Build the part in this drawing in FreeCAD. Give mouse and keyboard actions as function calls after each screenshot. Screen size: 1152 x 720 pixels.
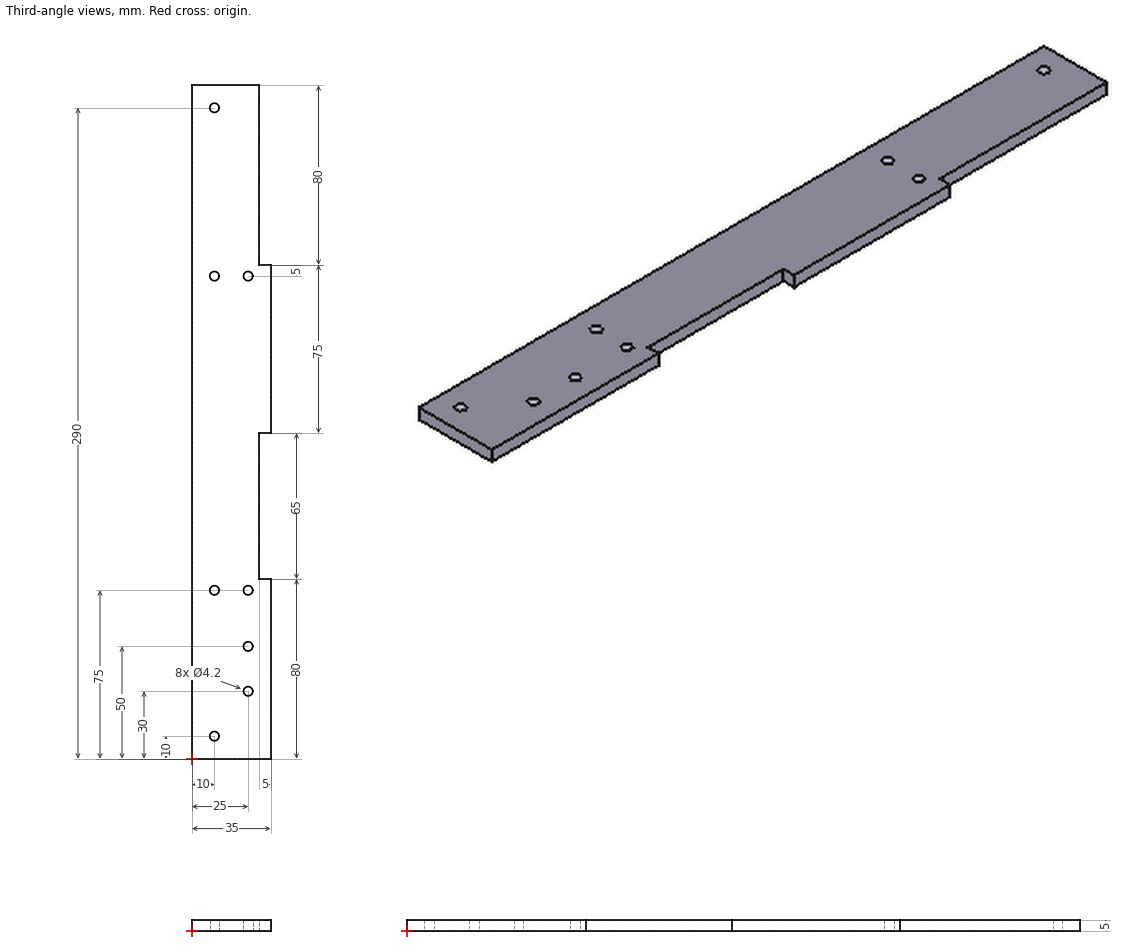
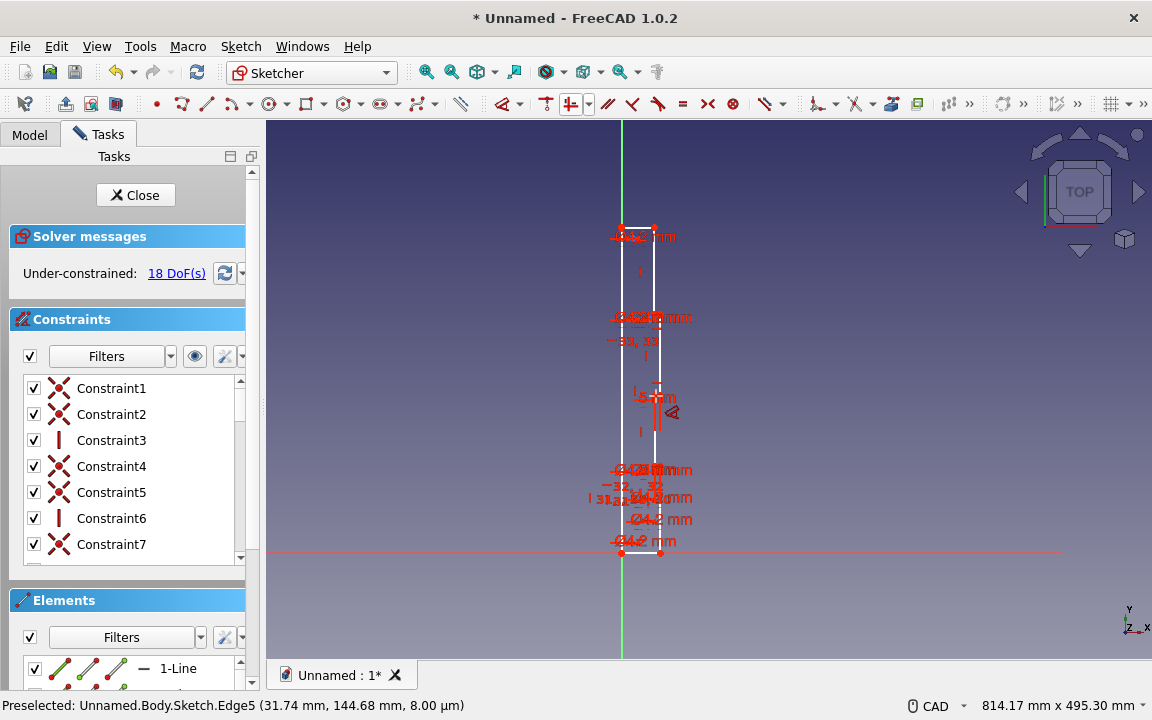
scroll(658, 315, up, 11)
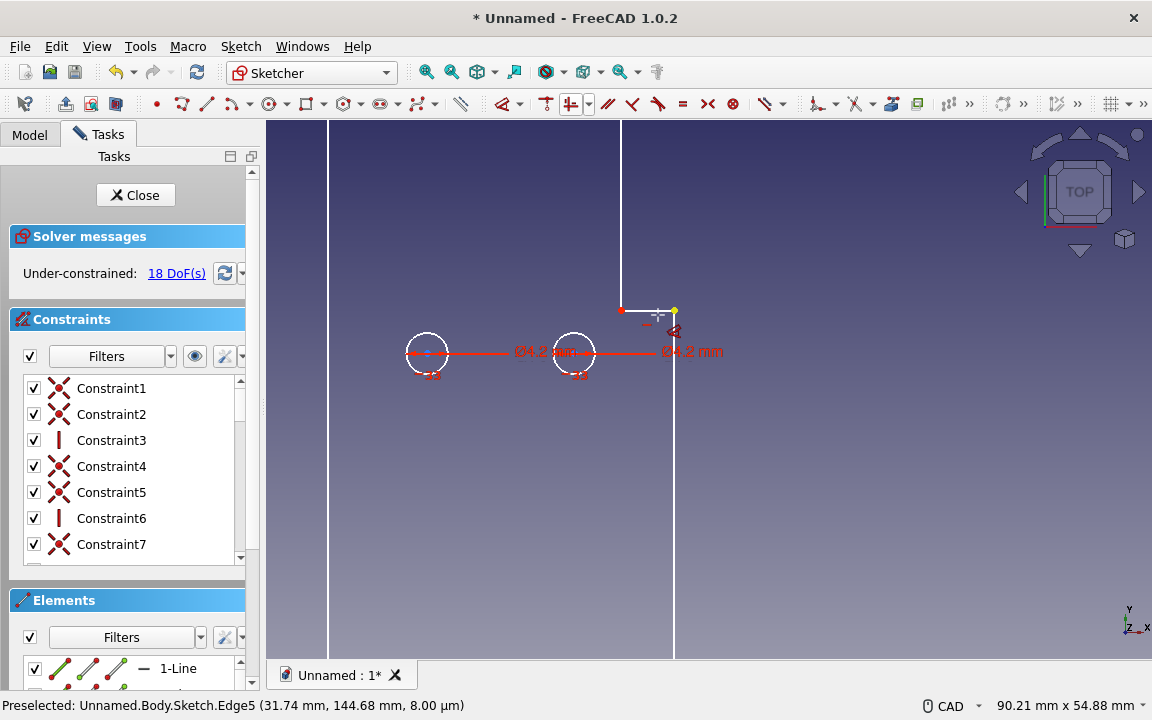
click(658, 311)
click(648, 277)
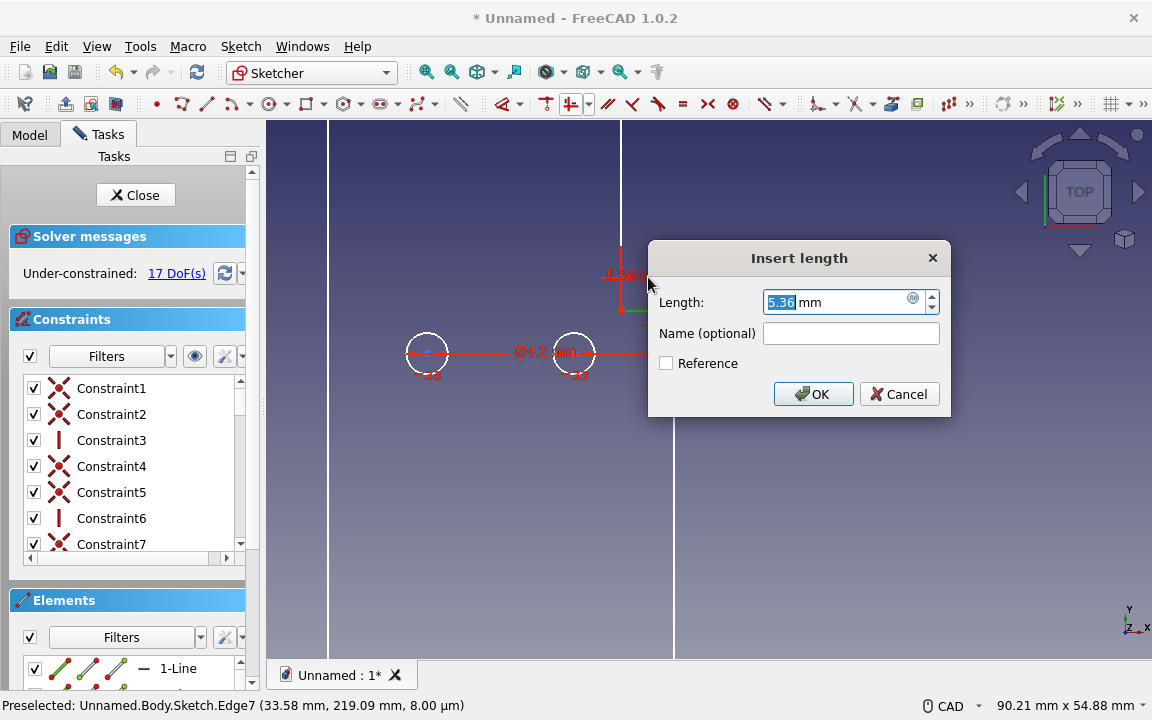
text(5)
key(Return)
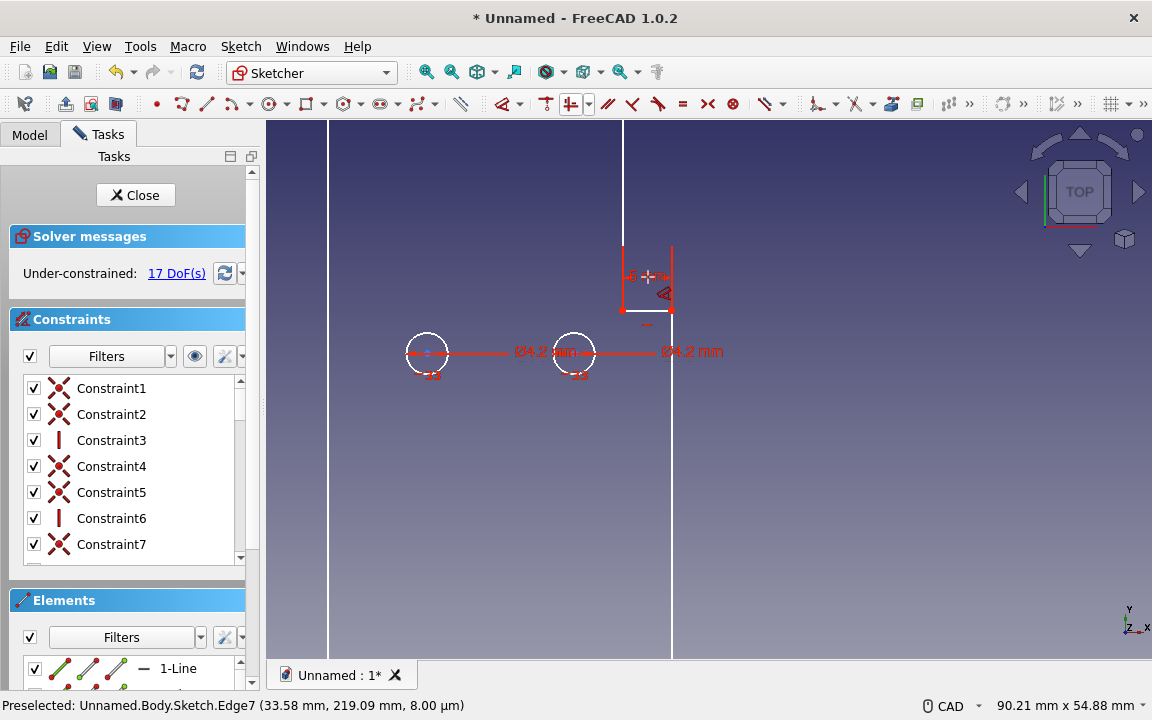
scroll(658, 315, down, 11)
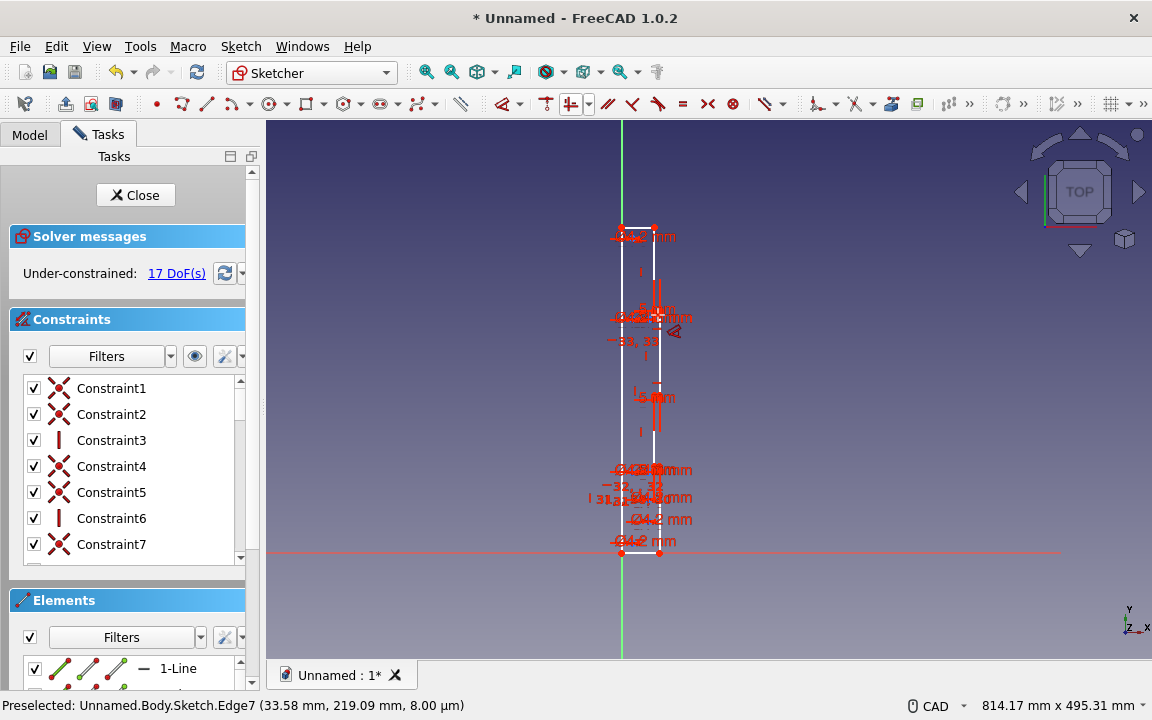
scroll(633, 553, up, 3)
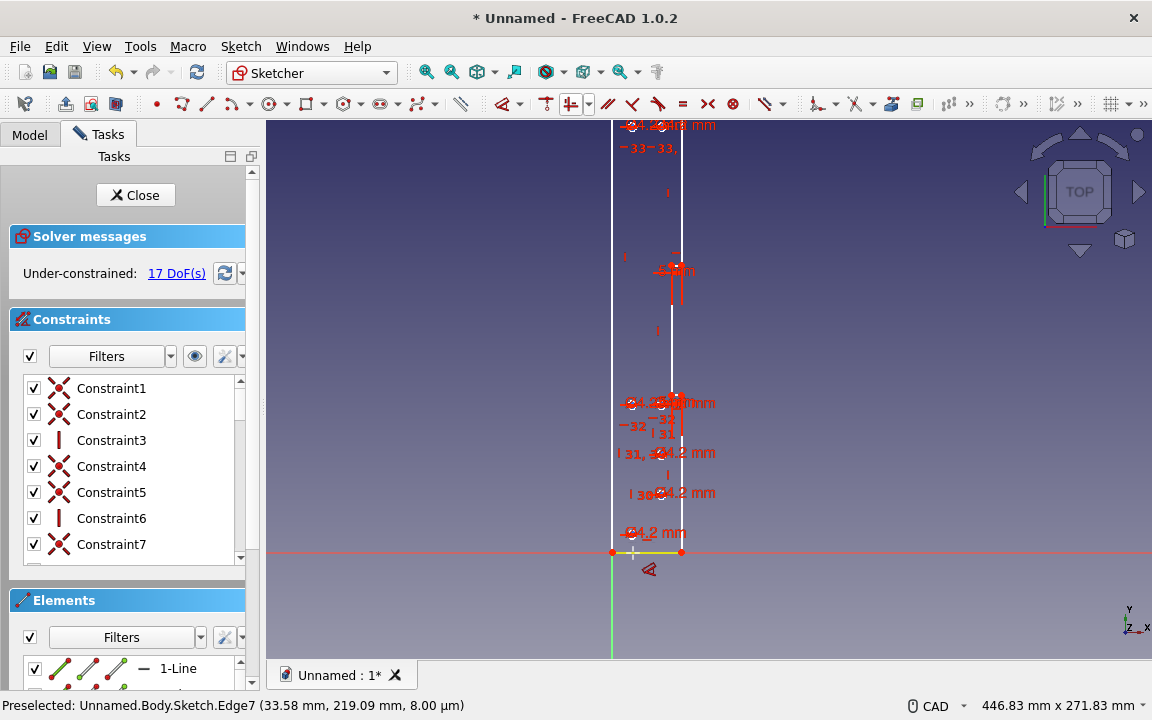
click(633, 553)
click(647, 587)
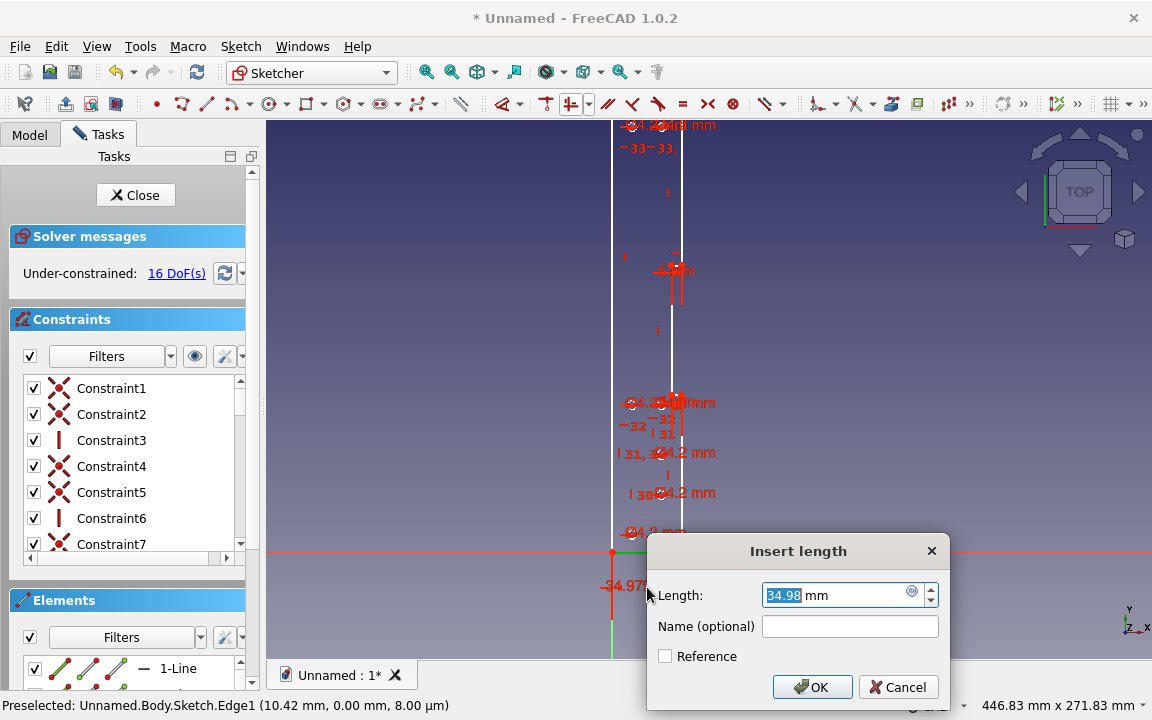
text(35)
key(Return)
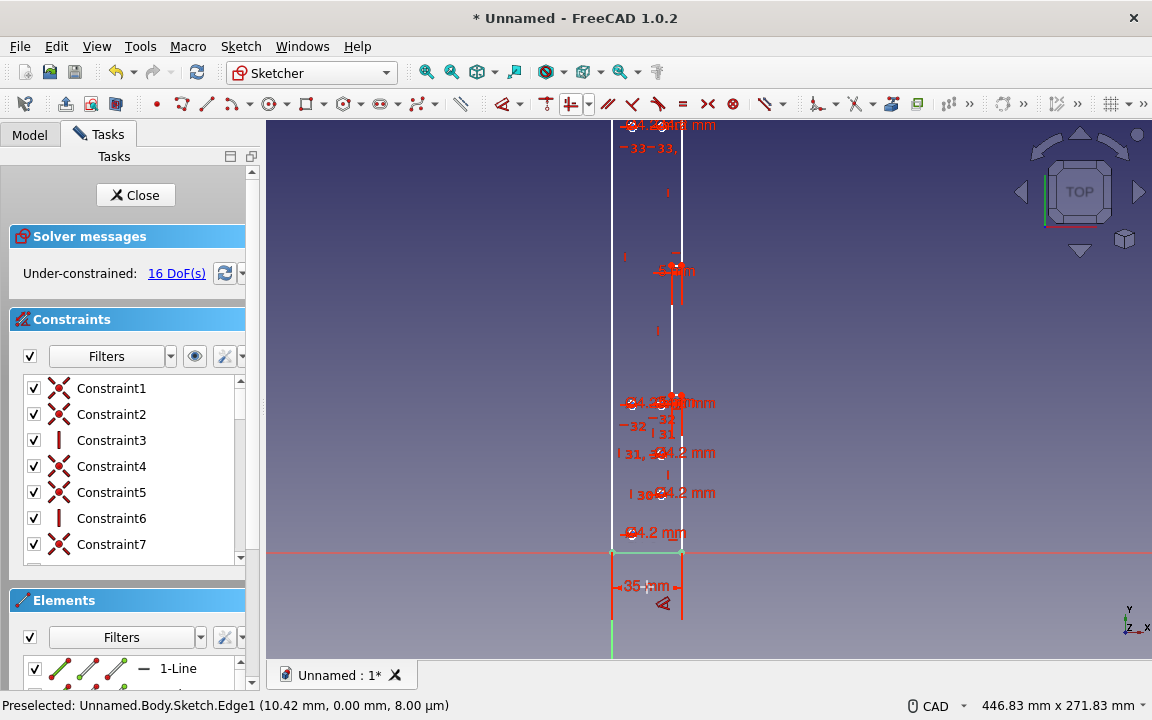
click(682, 506)
click(716, 474)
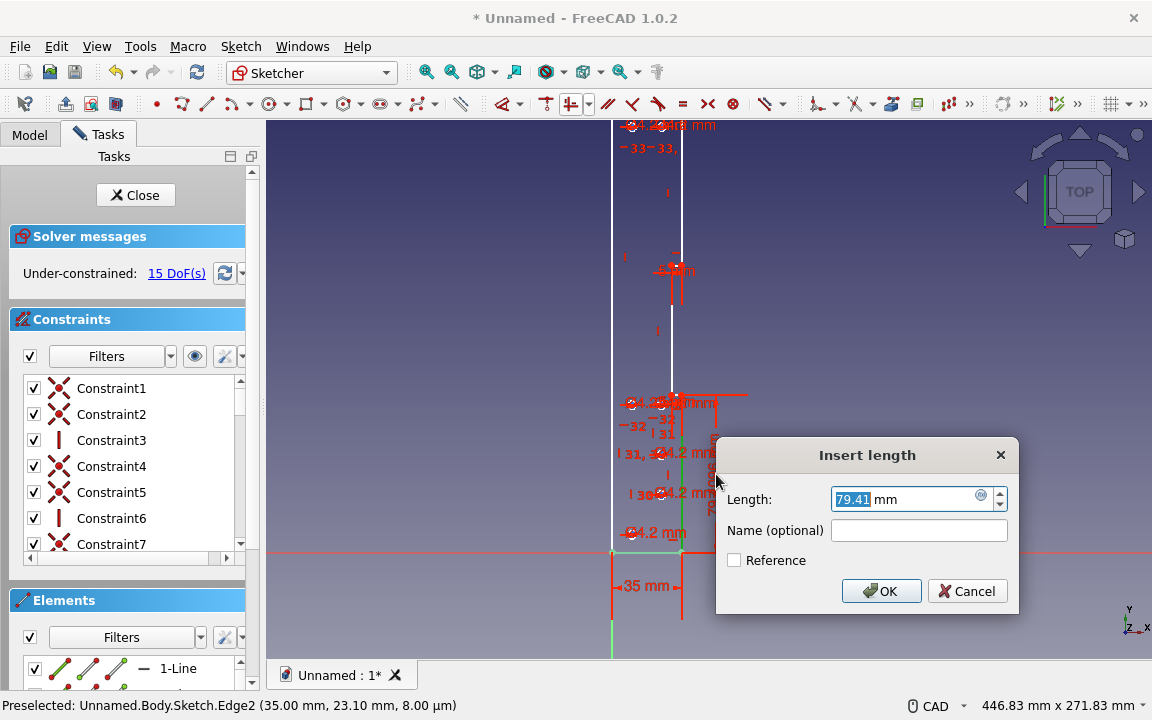
text(80)
key(Return)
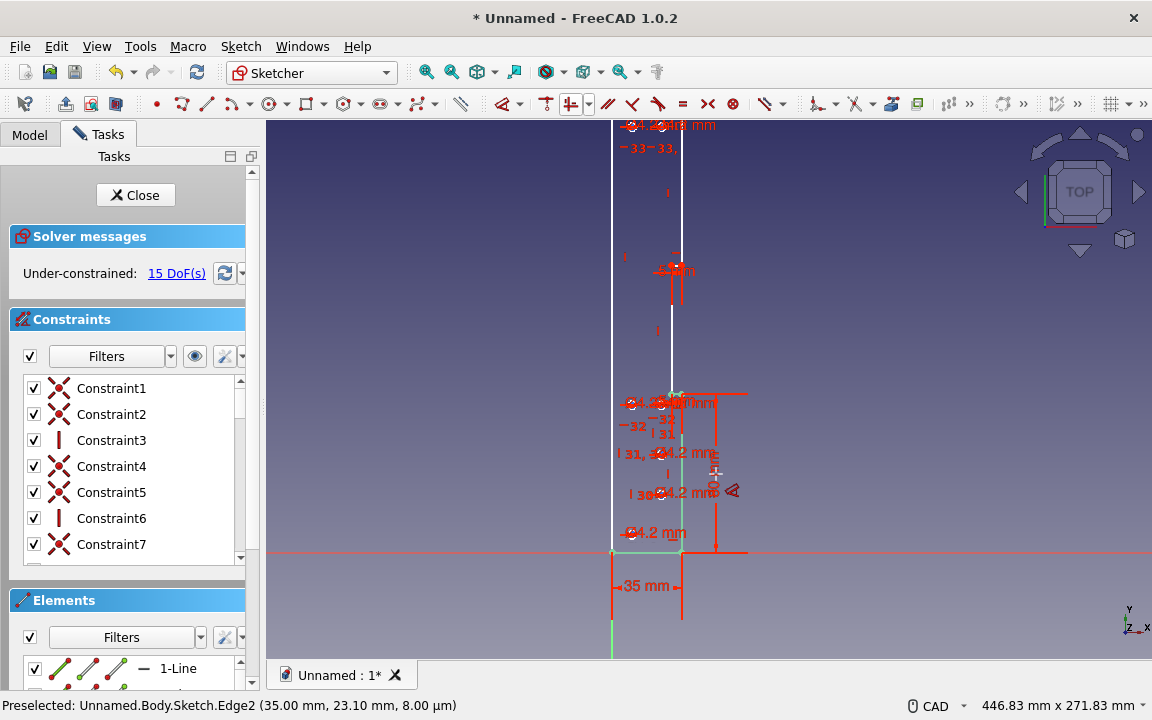
click(672, 356)
click(706, 330)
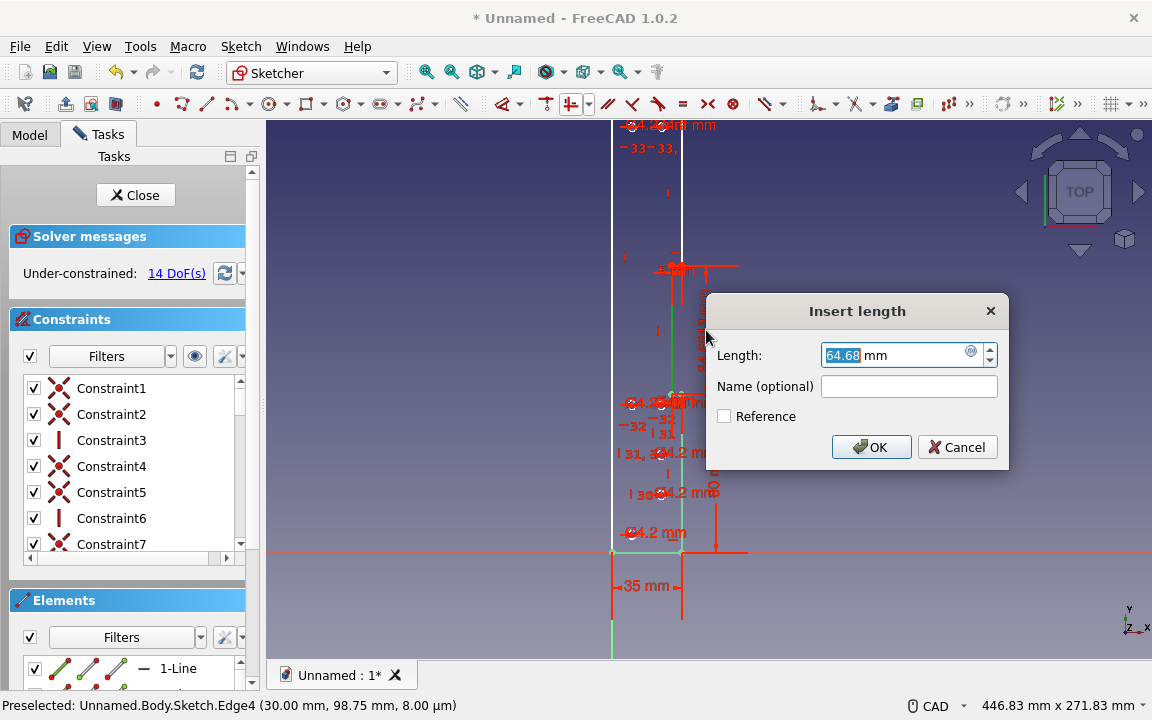
text(65)
key(Return)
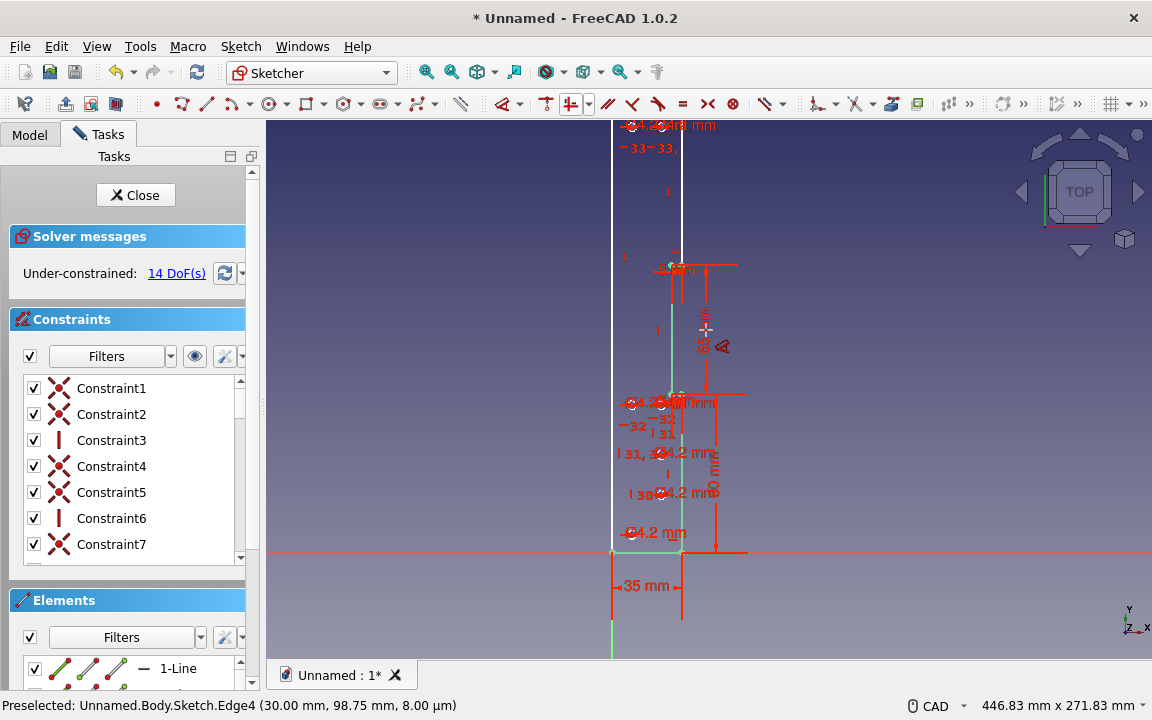
click(682, 221)
click(716, 207)